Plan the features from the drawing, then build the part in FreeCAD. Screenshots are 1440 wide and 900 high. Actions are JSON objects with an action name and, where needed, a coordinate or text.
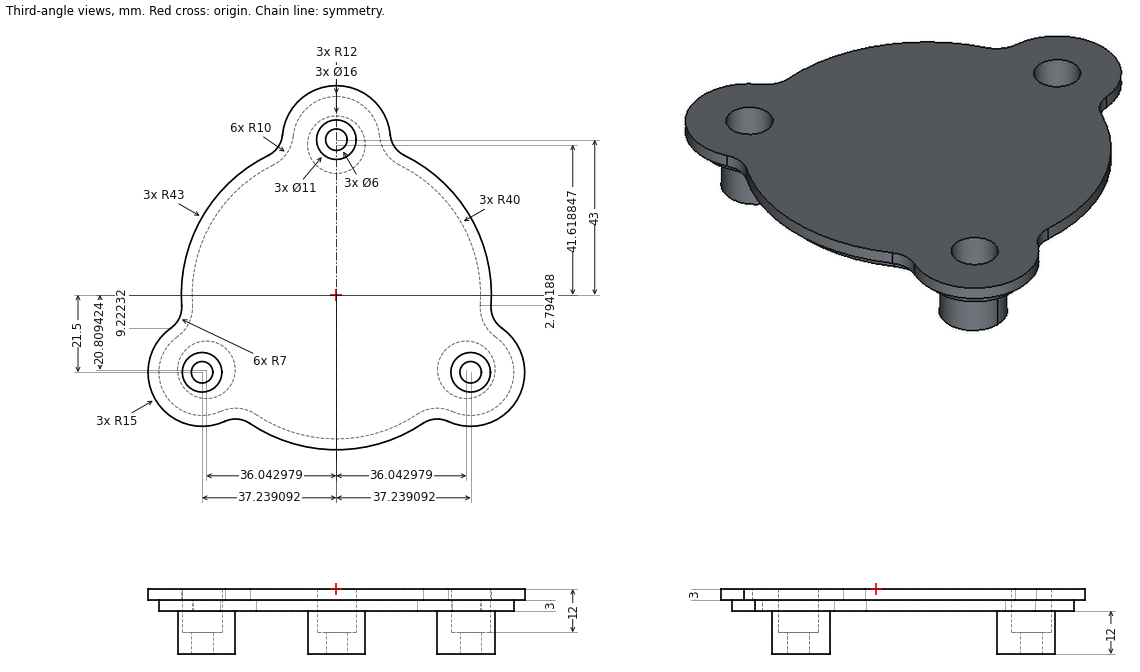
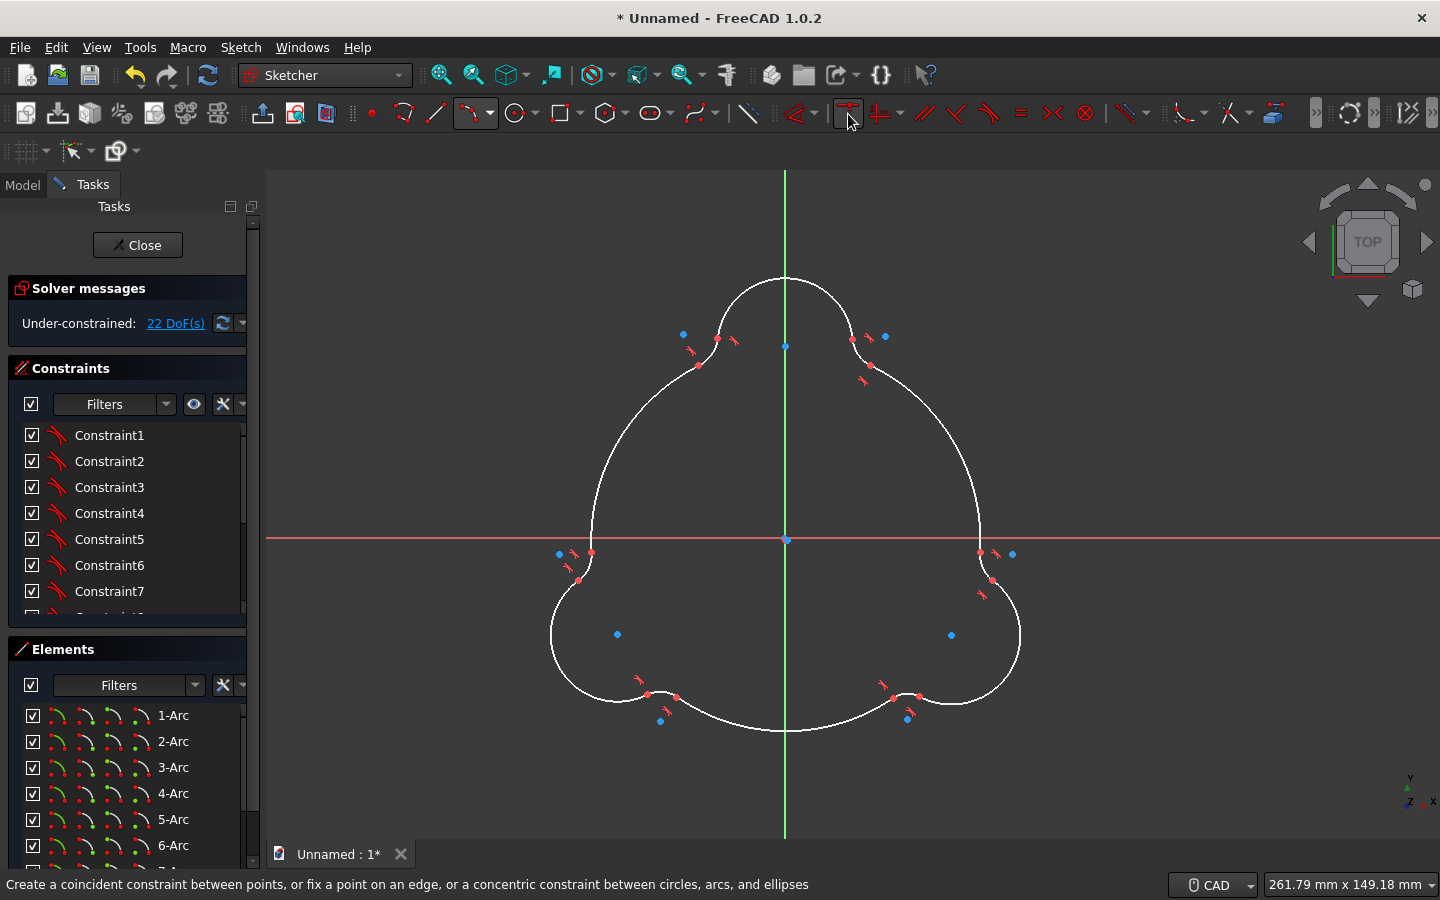
{"action": "left_click", "coordinate": [739, 725]}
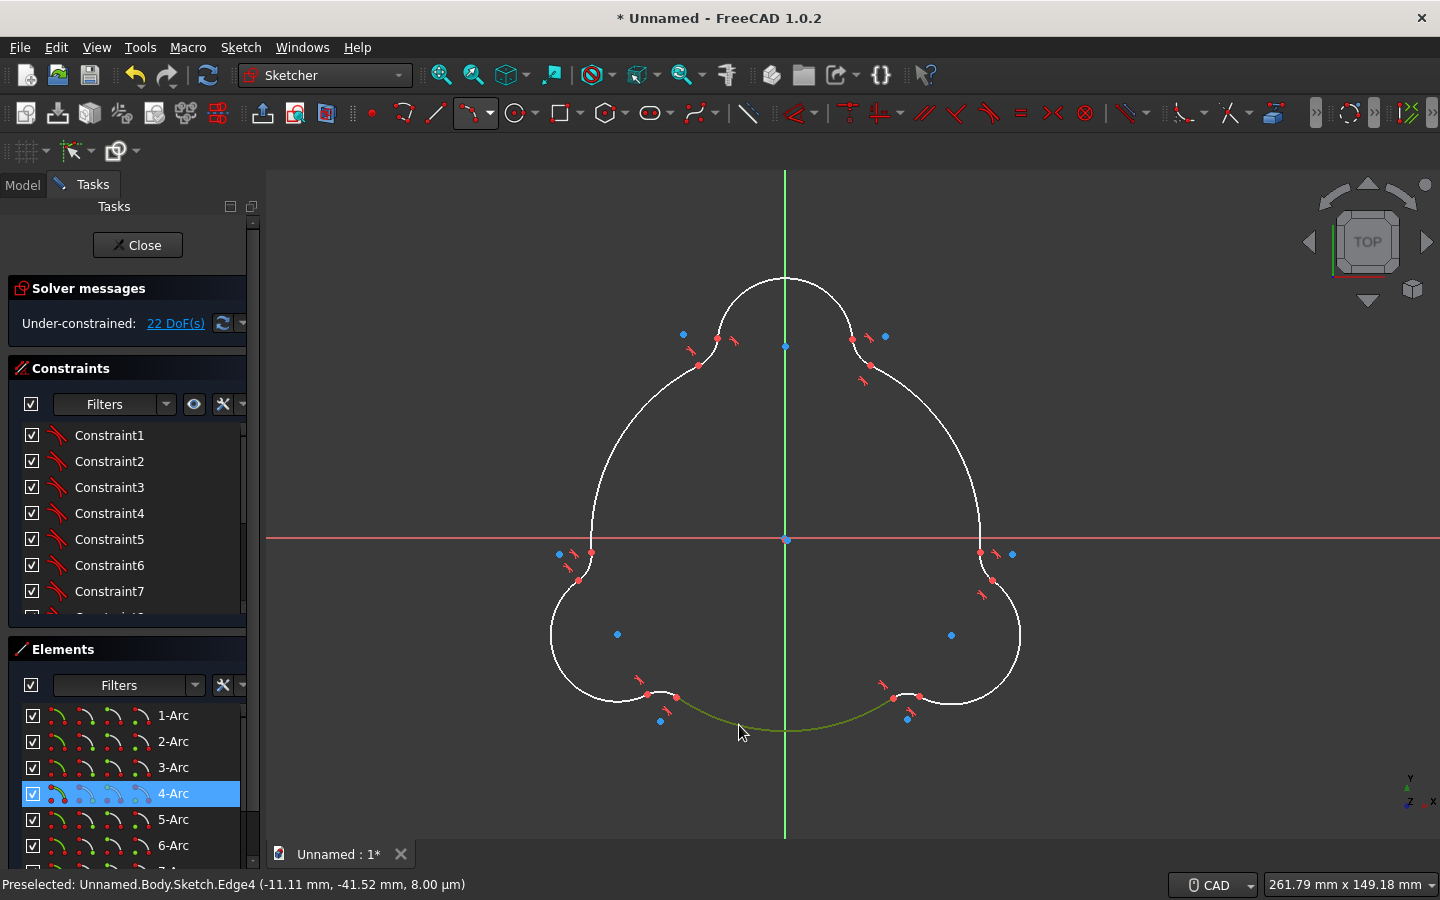
{"action": "left_click", "coordinate": [644, 406]}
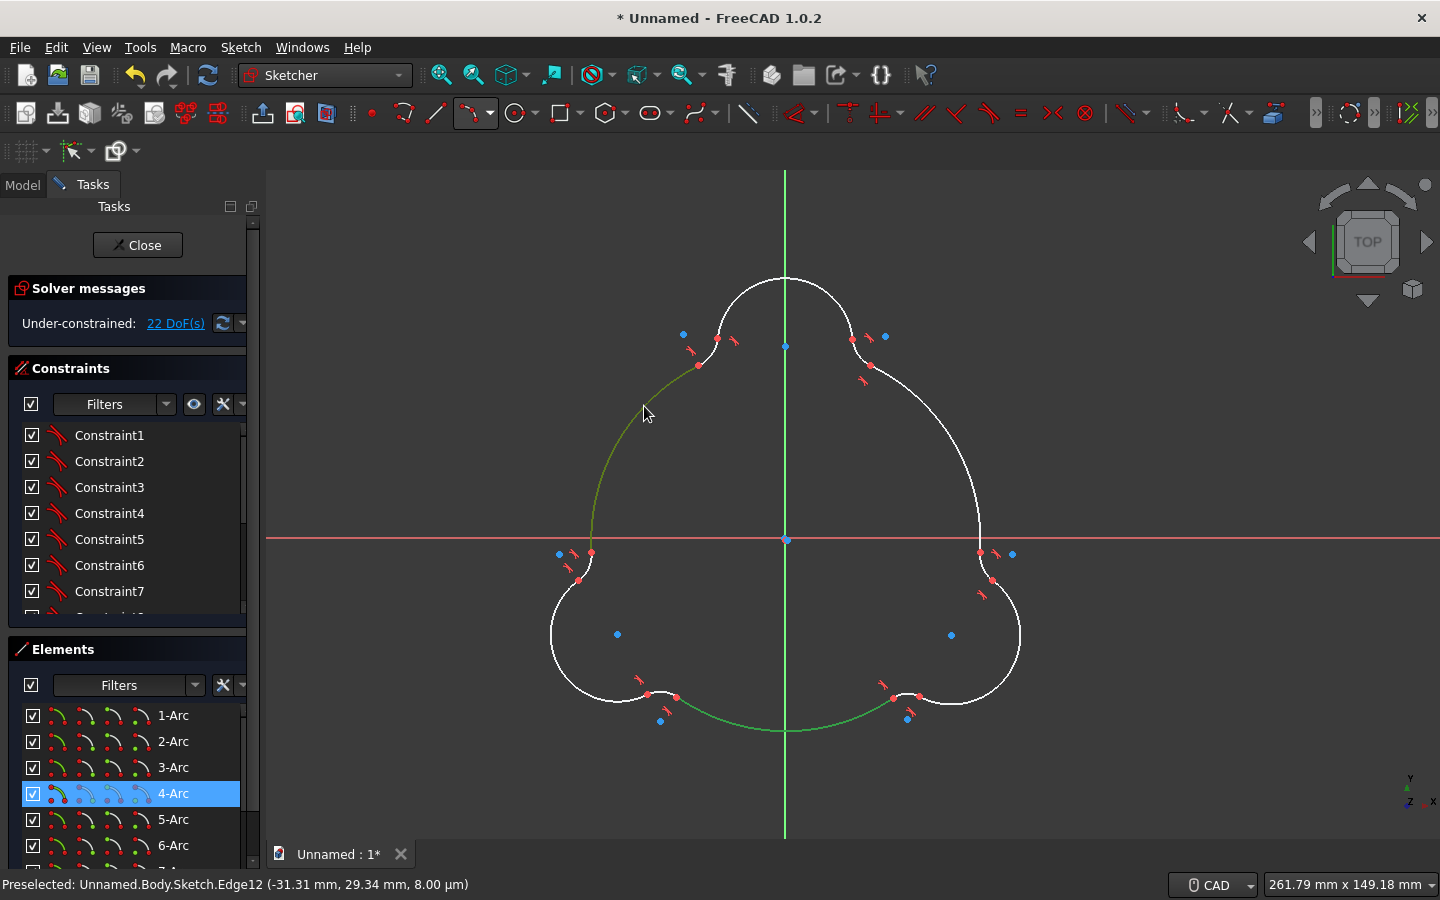
{"action": "left_click", "coordinate": [848, 114]}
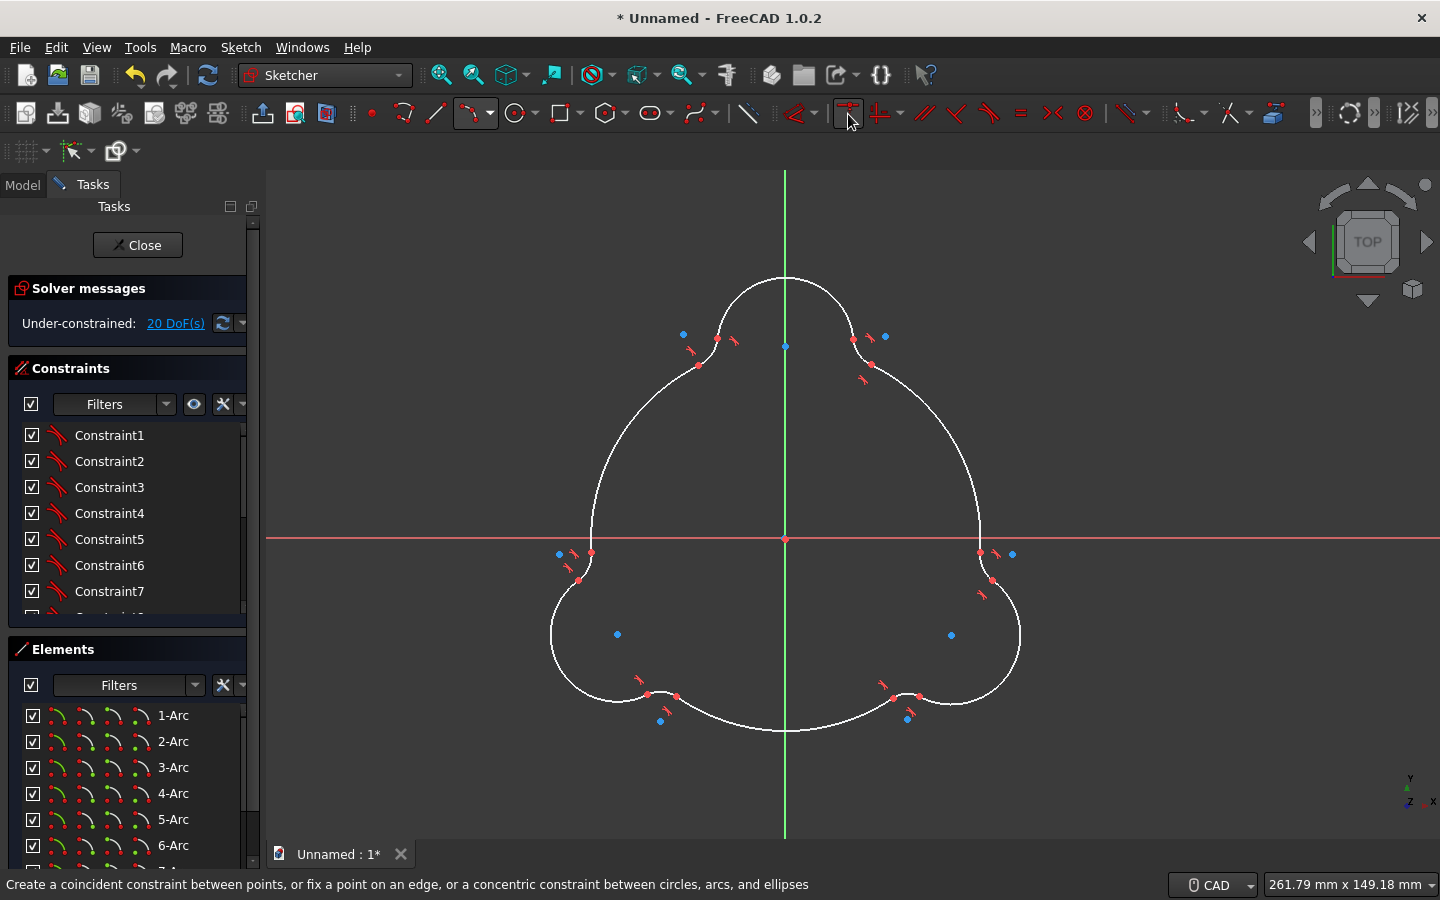
{"action": "scroll", "coordinate": [785, 539], "scroll_direction": "up", "scroll_amount": 3}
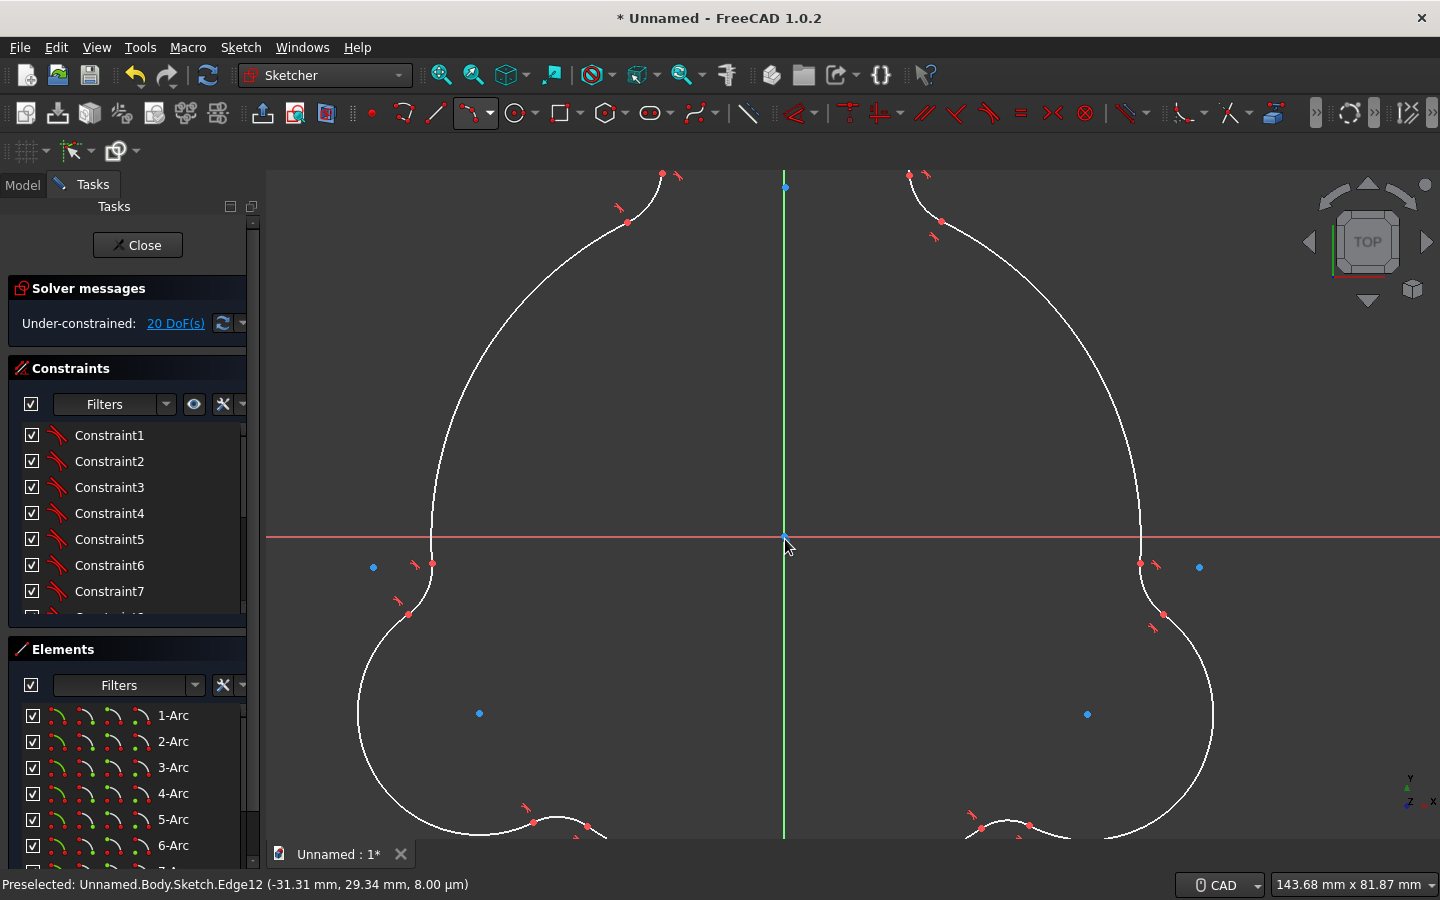
{"action": "left_click_drag", "start_coordinate": [774, 527], "coordinate": [796, 550]}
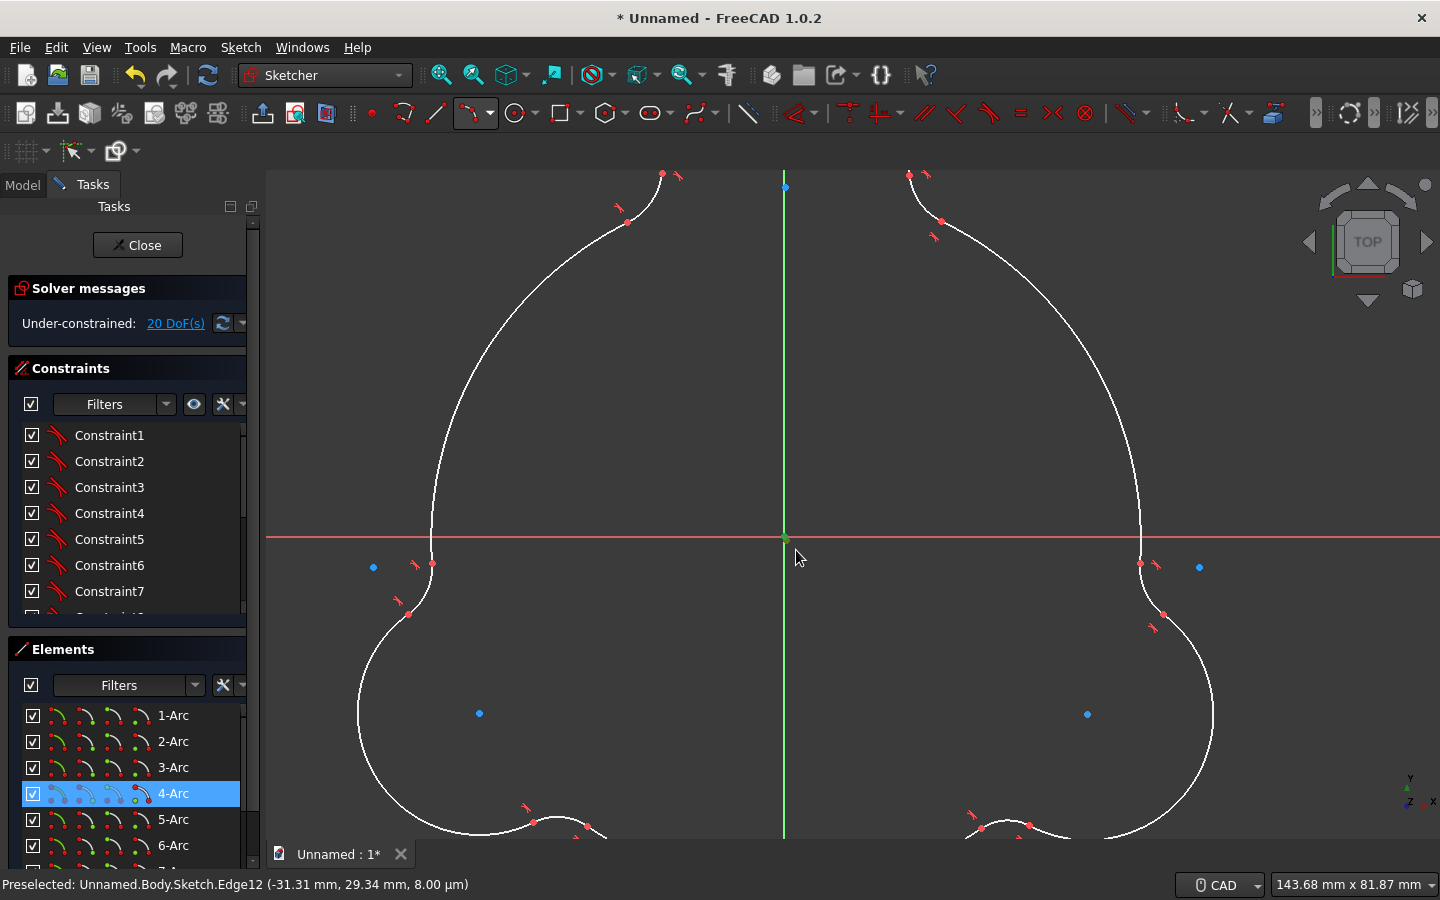
{"action": "left_click", "coordinate": [848, 114]}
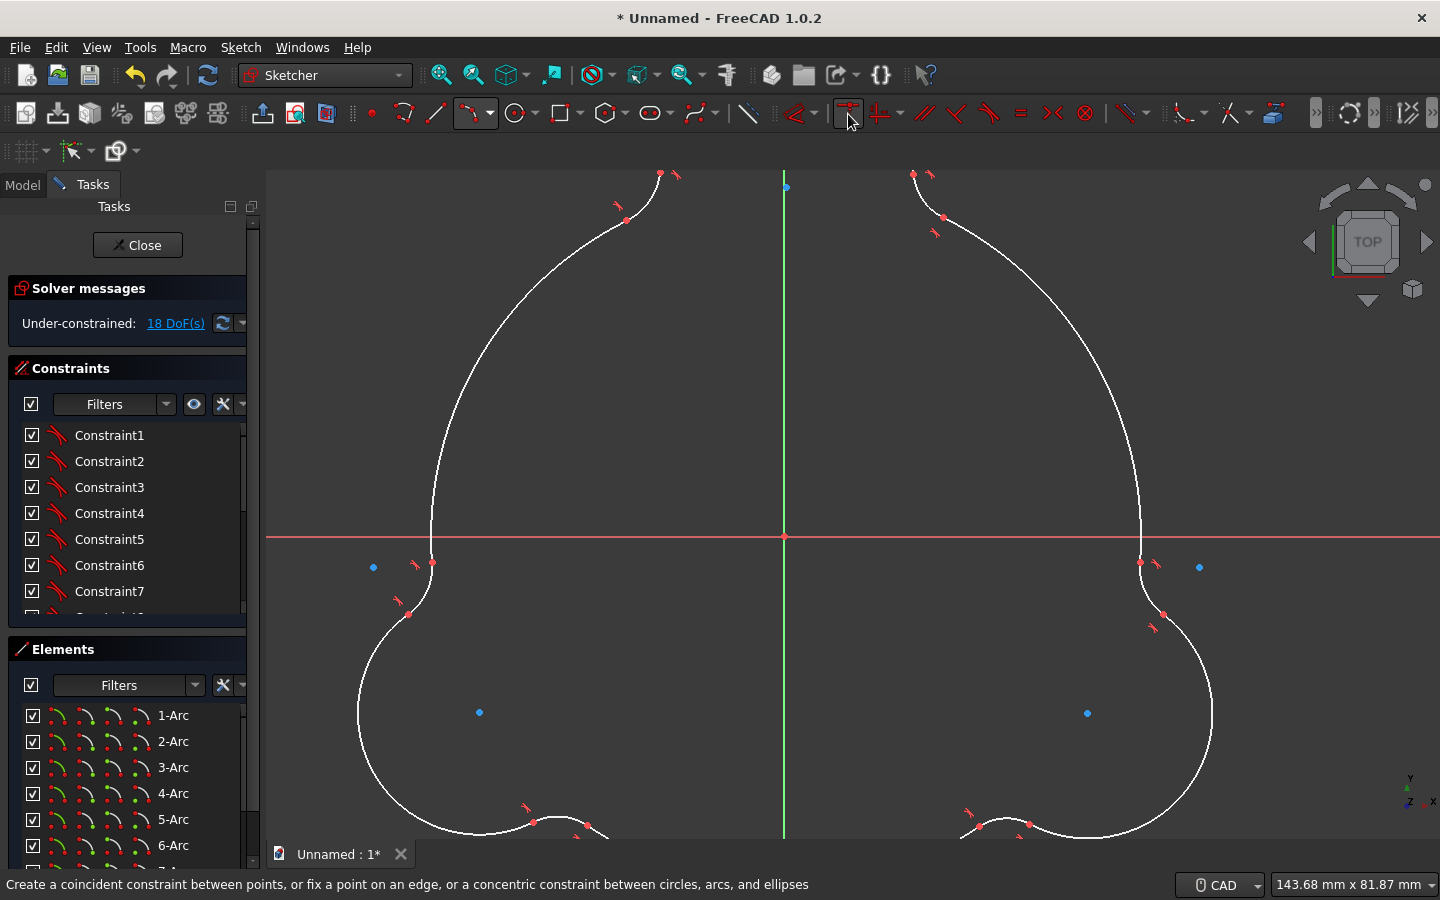
{"action": "left_click", "coordinate": [421, 602]}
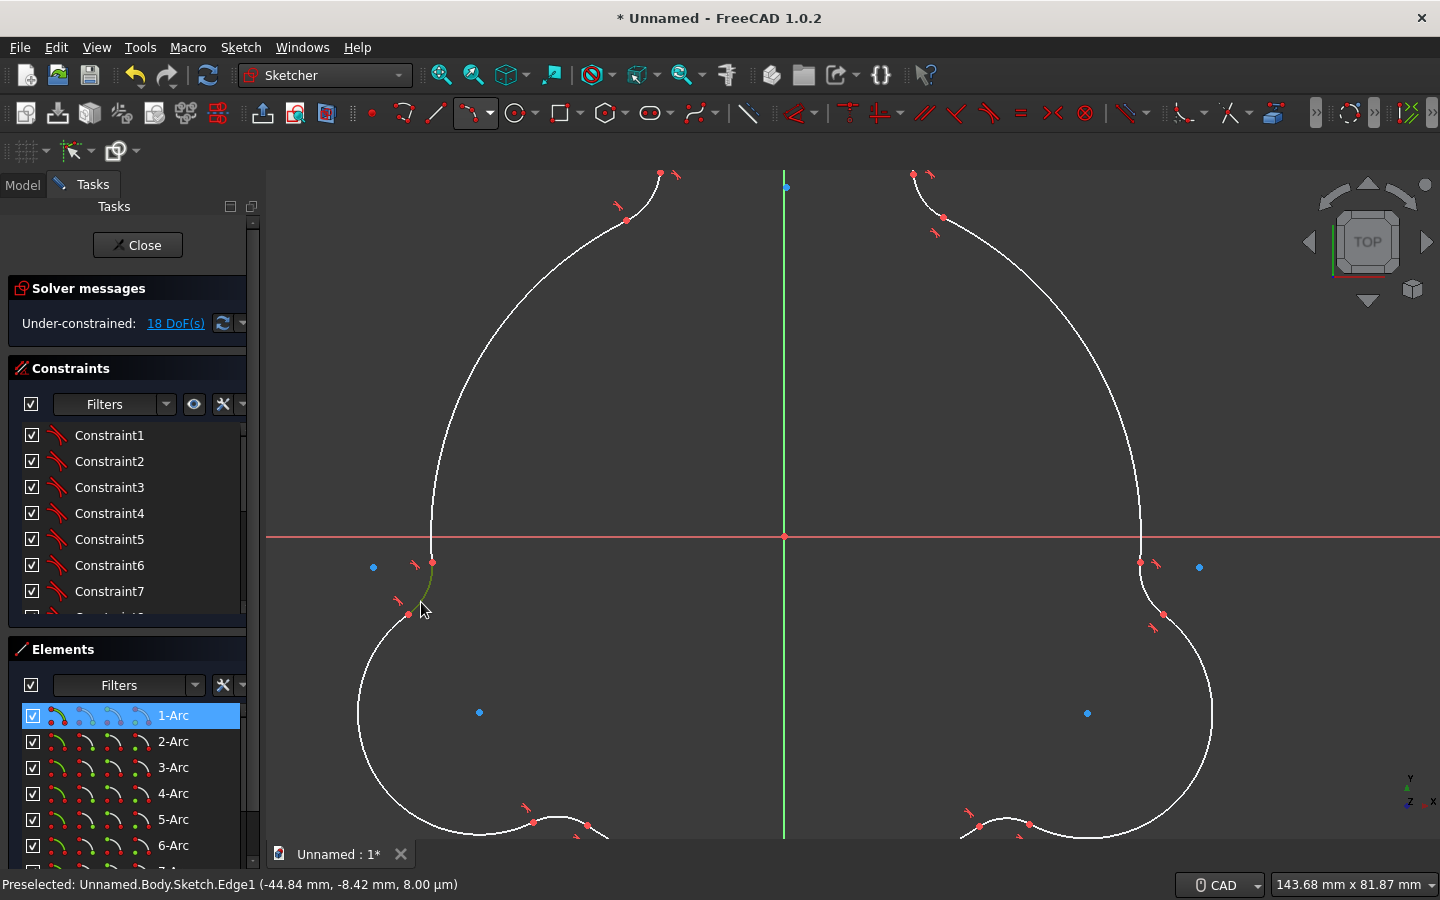
{"action": "scroll", "coordinate": [785, 540], "scroll_direction": "down", "scroll_amount": 3}